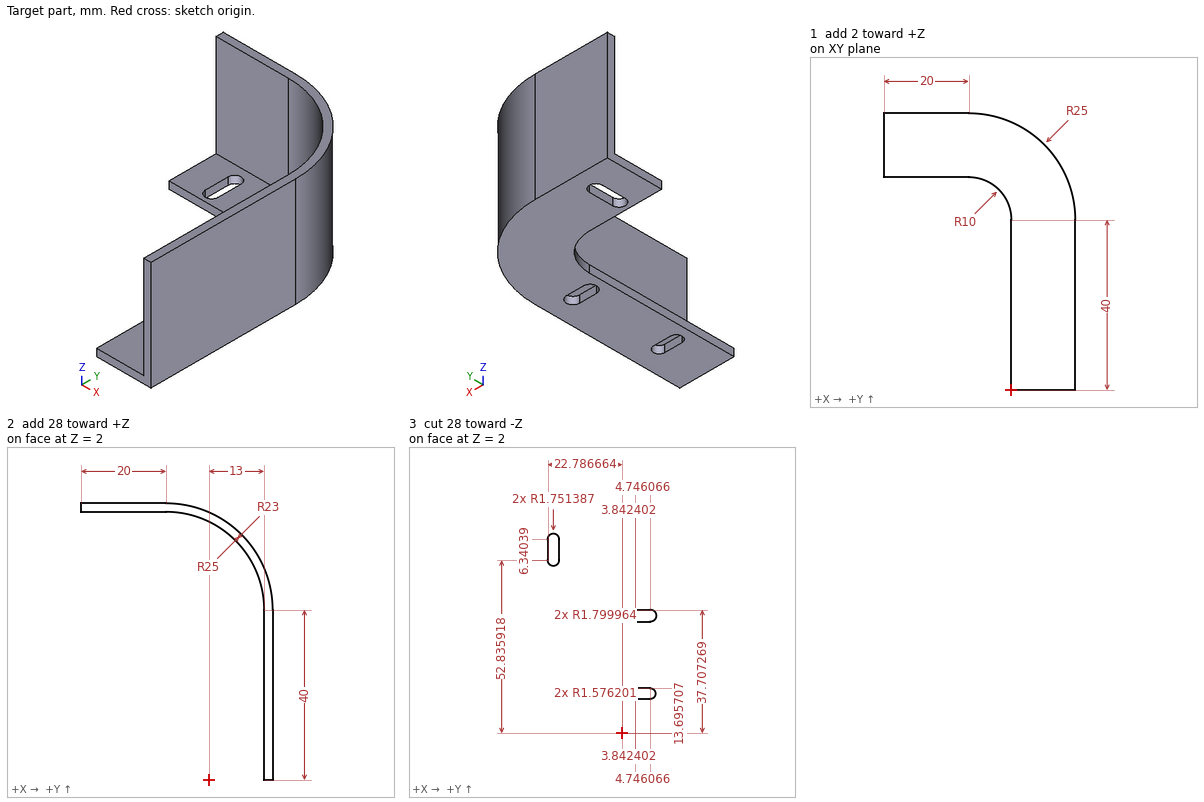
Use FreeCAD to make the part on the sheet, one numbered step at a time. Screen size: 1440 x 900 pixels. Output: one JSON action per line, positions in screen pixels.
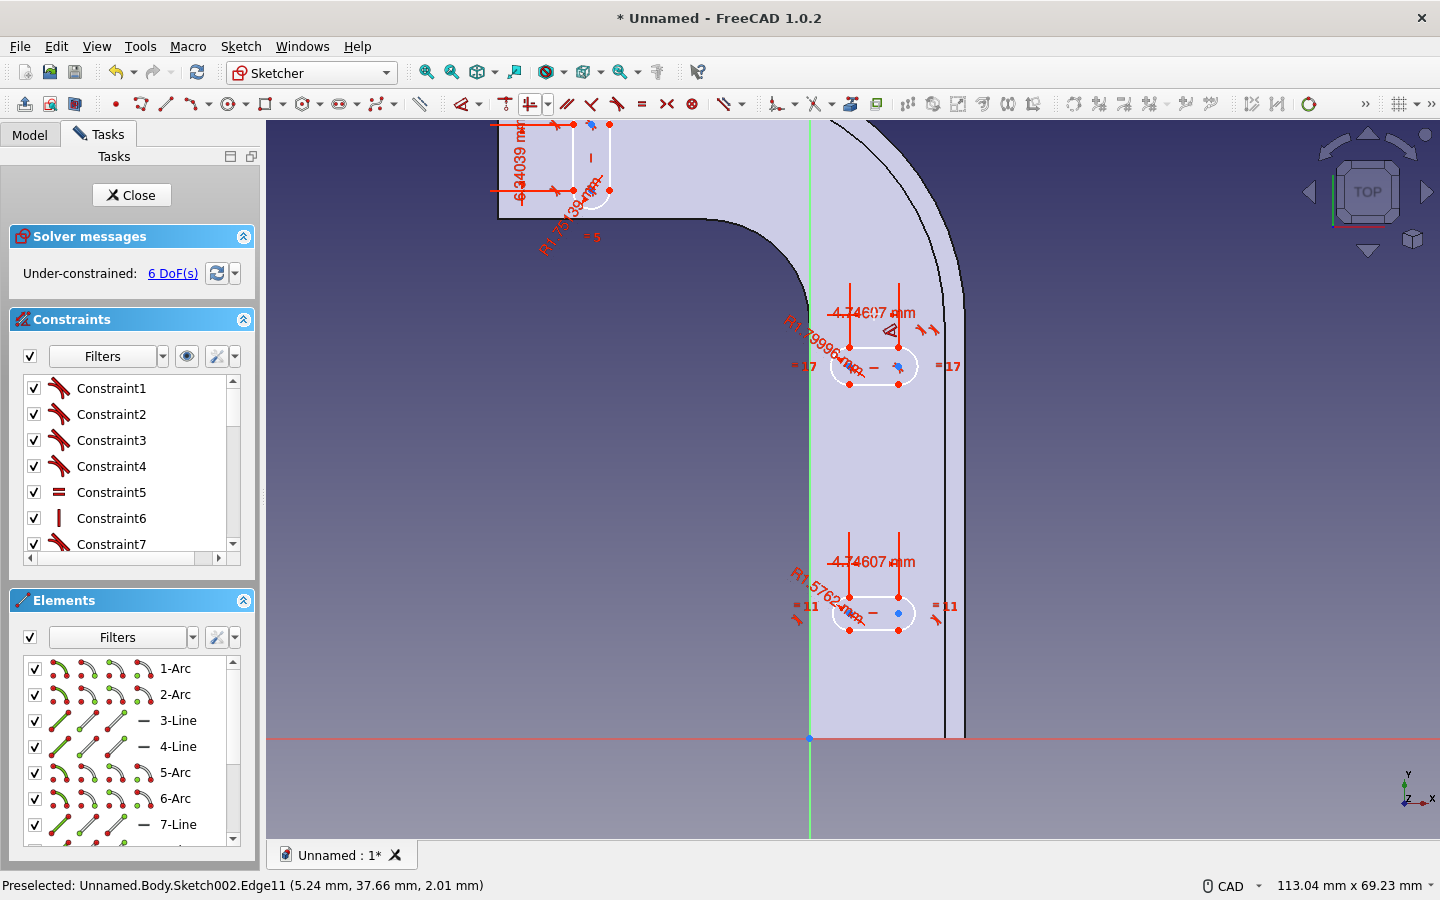
{"action": "left_click", "coordinate": [849, 597]}
{"action": "left_click", "coordinate": [829, 773]}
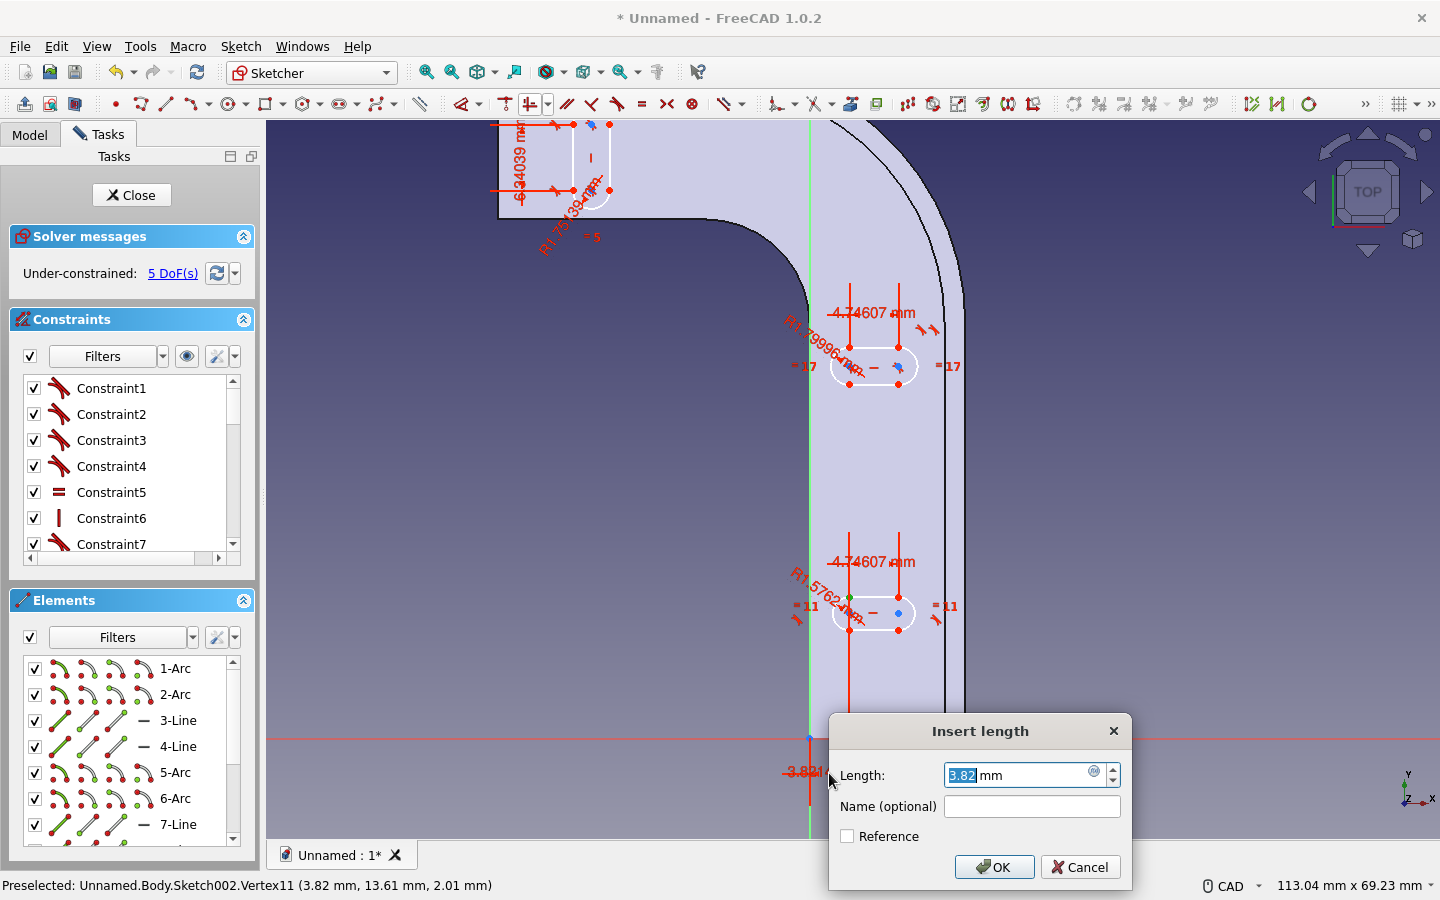
{"action": "type", "text": "3.842402"}
{"action": "key", "text": "Return"}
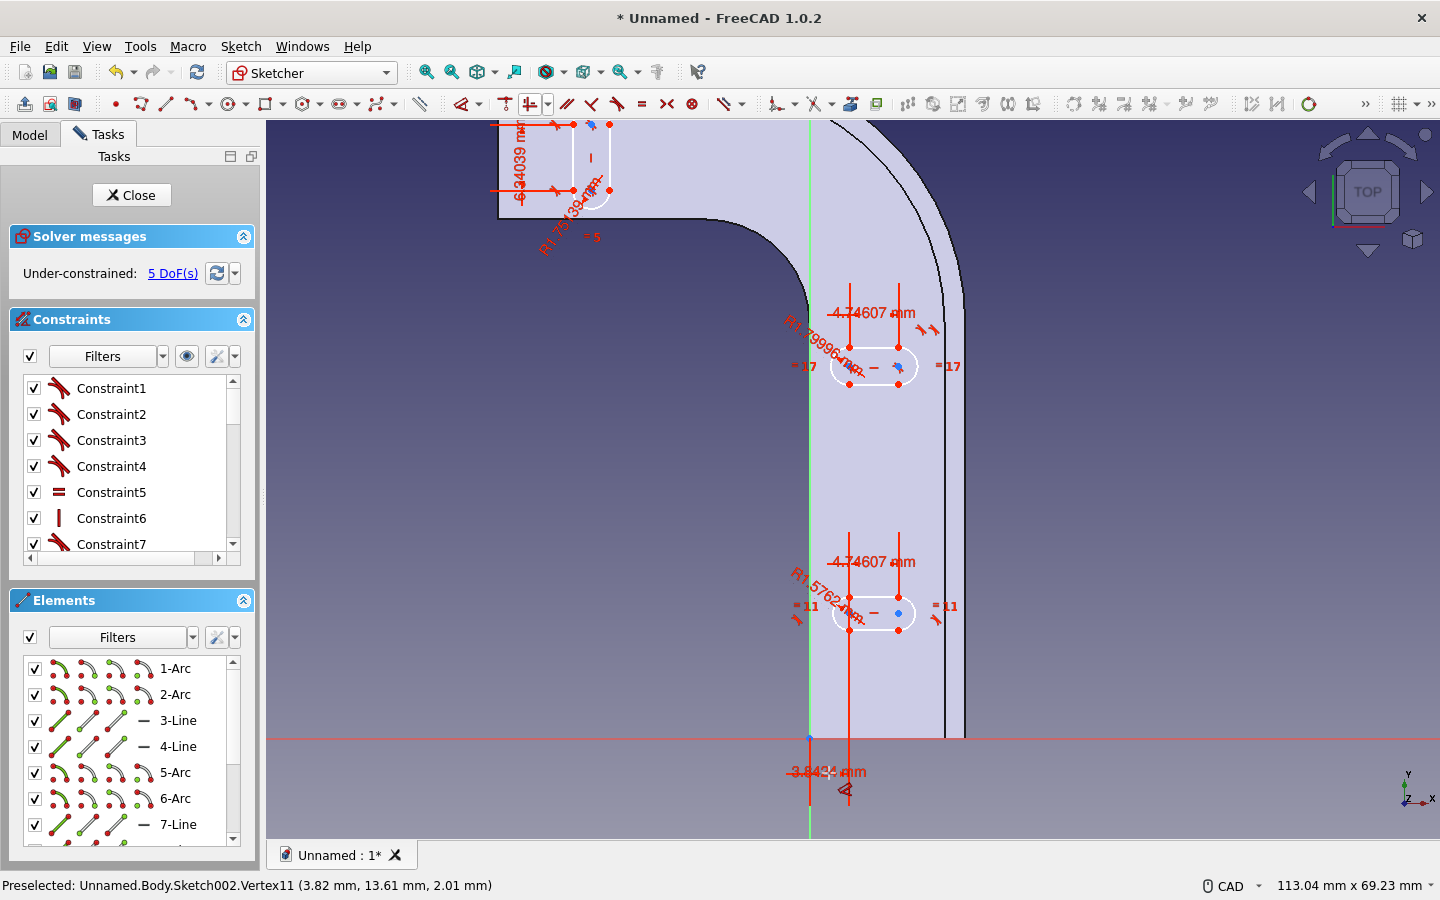
{"action": "left_click", "coordinate": [850, 348]}
{"action": "left_click", "coordinate": [830, 797]}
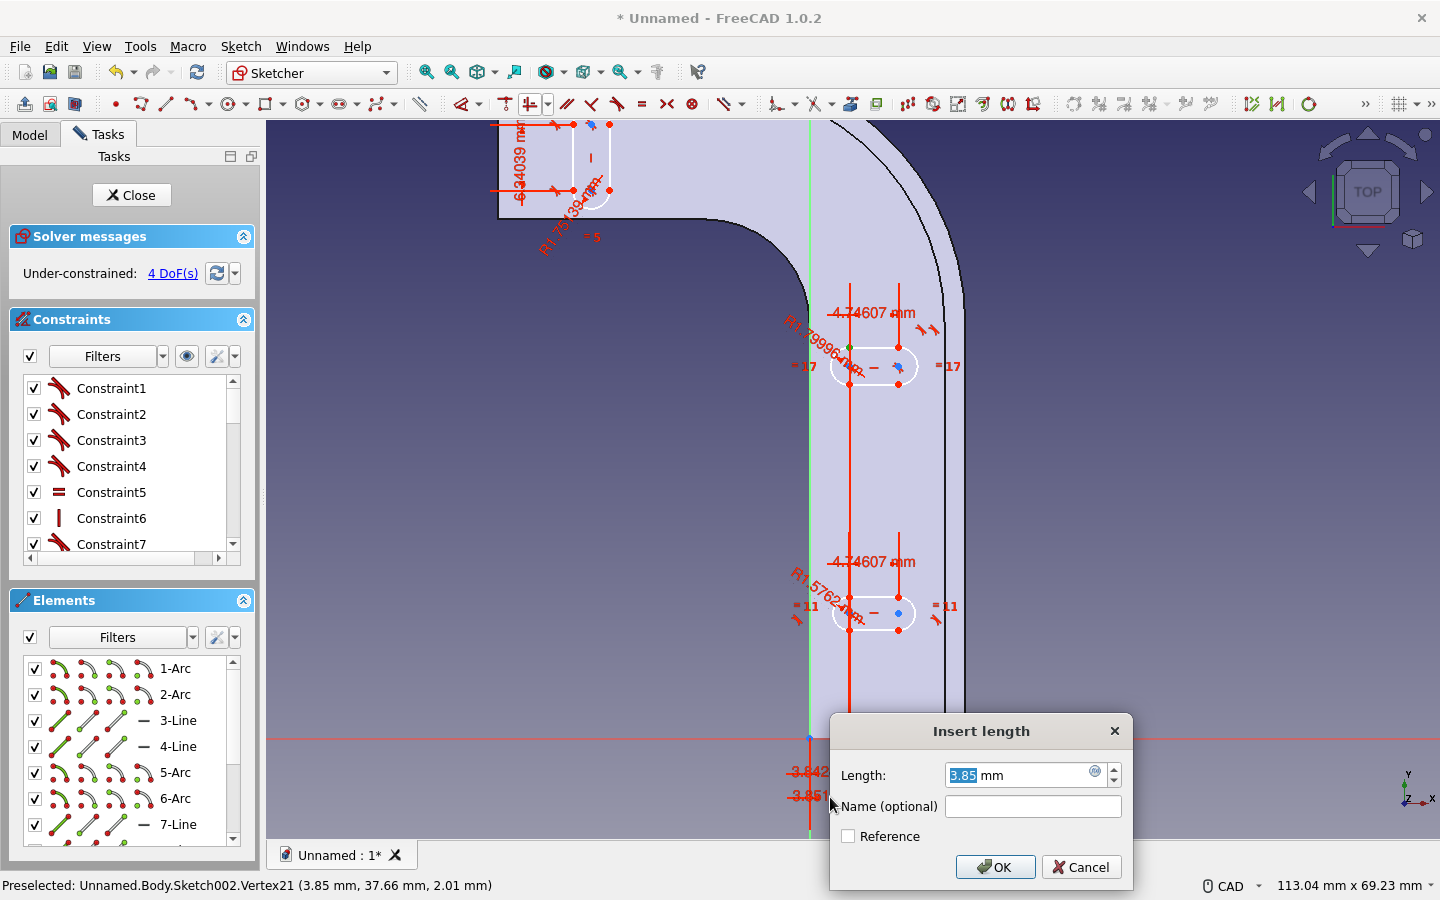
{"action": "type", "text": "3.842402"}
{"action": "key", "text": "Return"}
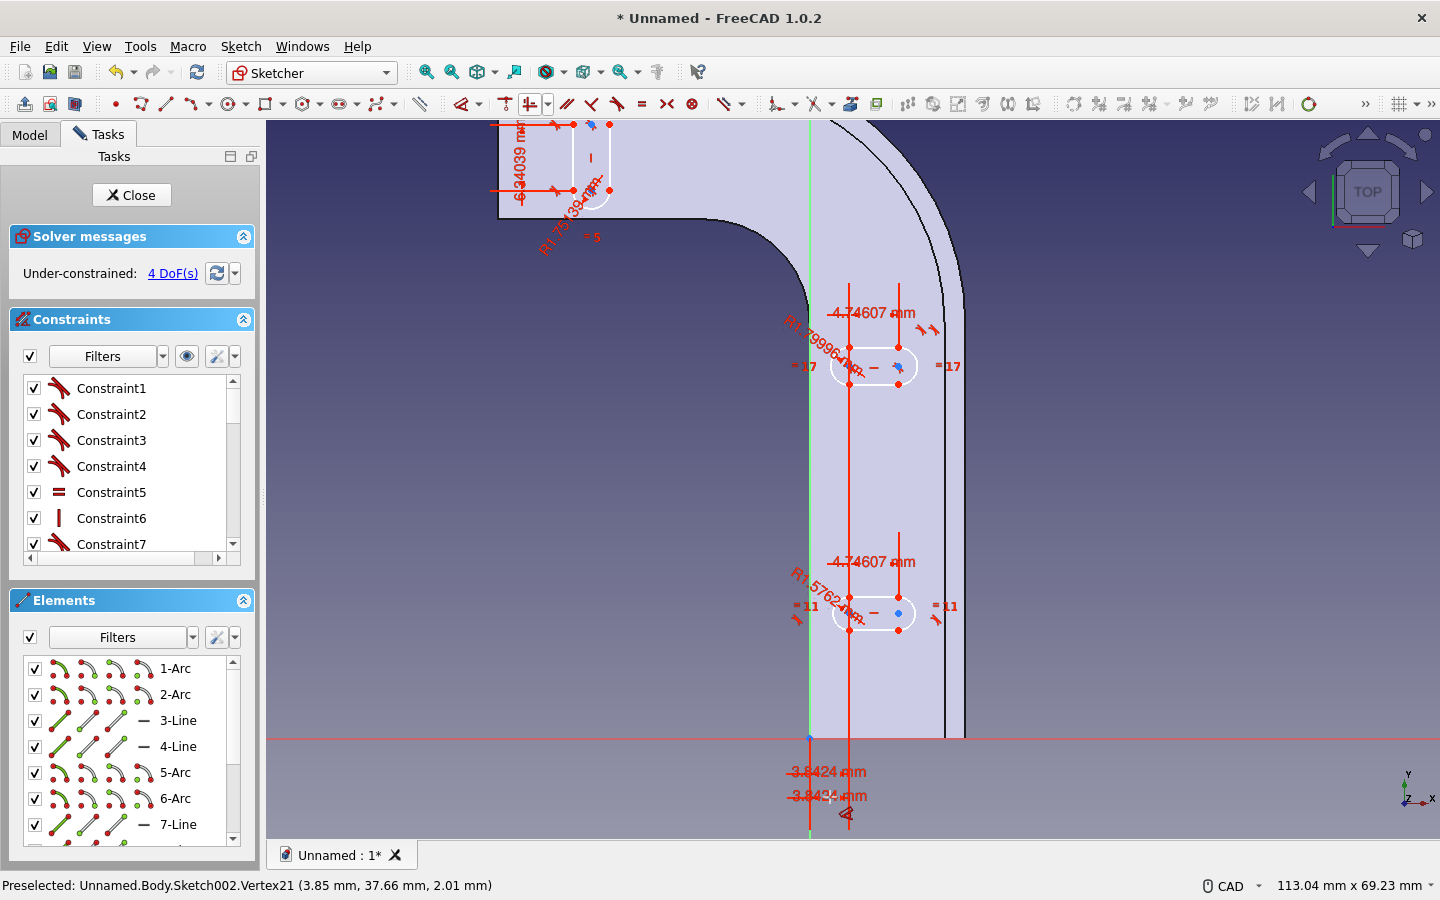
{"action": "left_click", "coordinate": [573, 191]}
{"action": "left_click", "coordinate": [691, 773]}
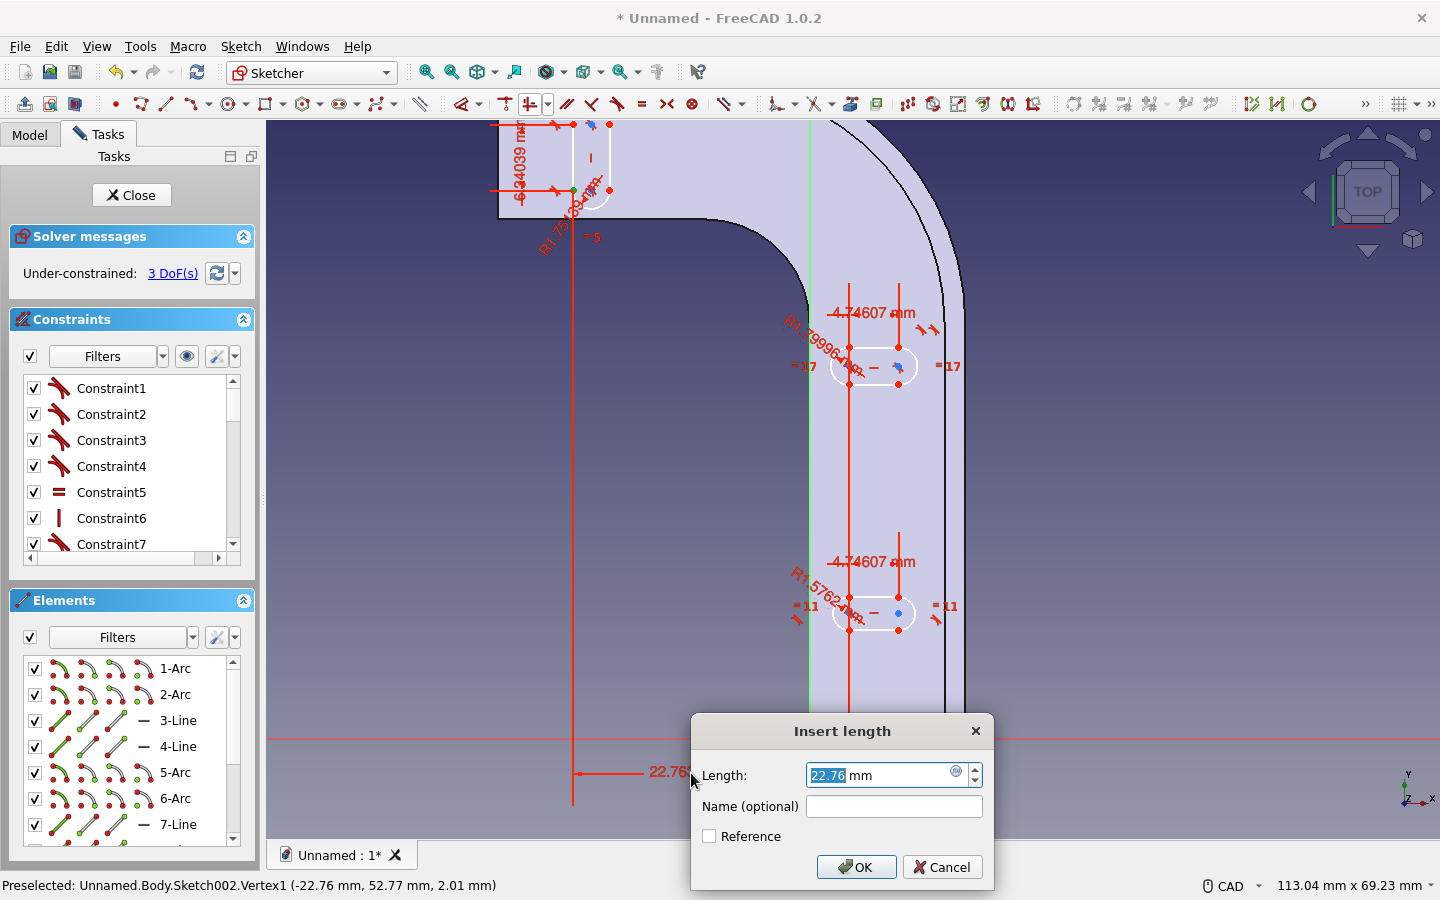
{"action": "type", "text": "22.786664"}
{"action": "key", "text": "Return"}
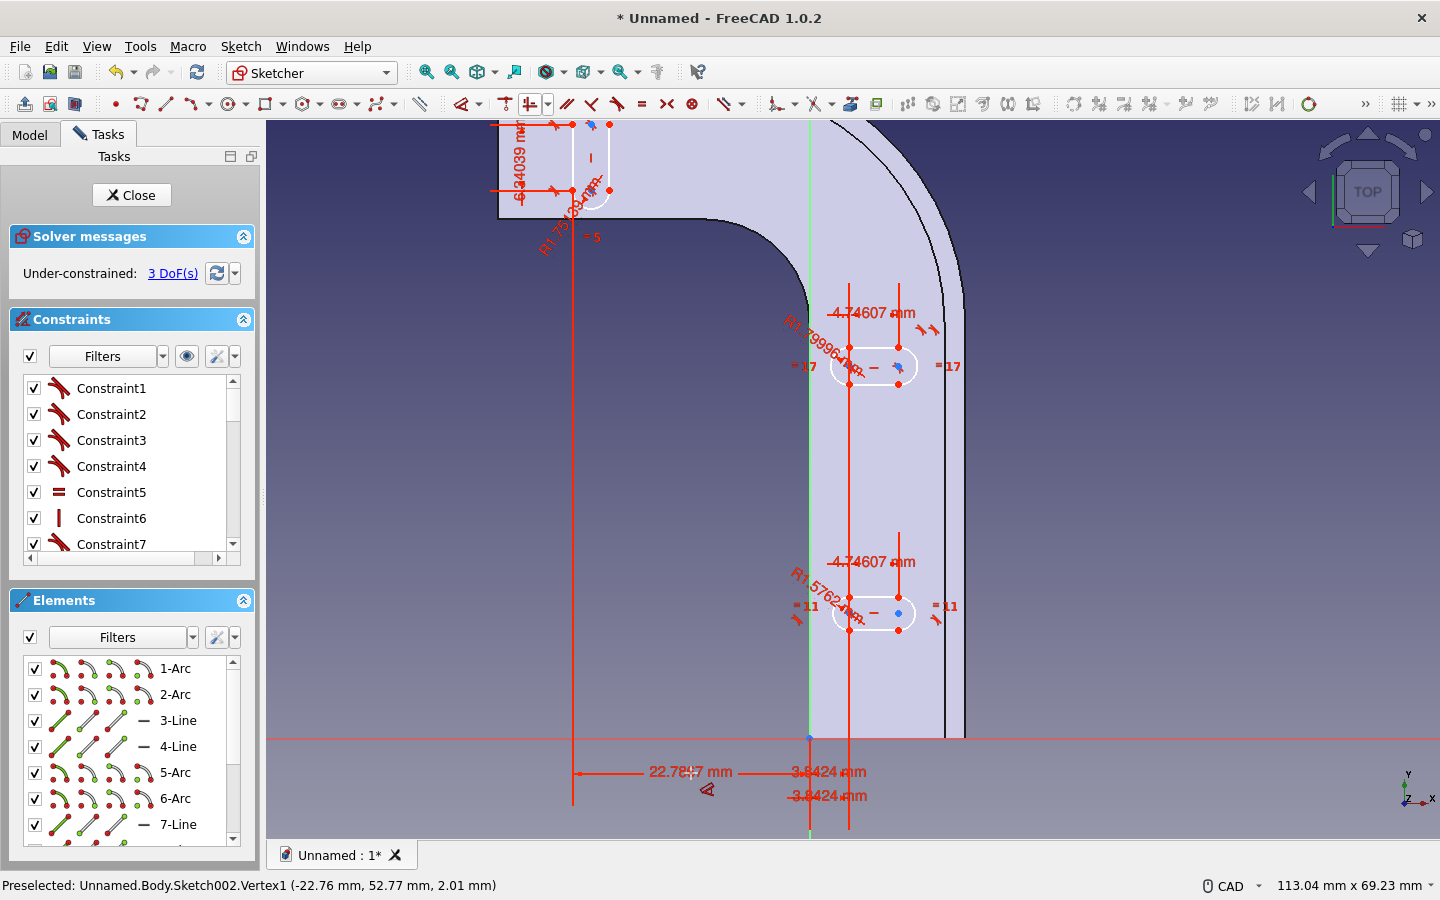
{"action": "left_click", "coordinate": [573, 191]}
{"action": "left_click", "coordinate": [539, 465]}